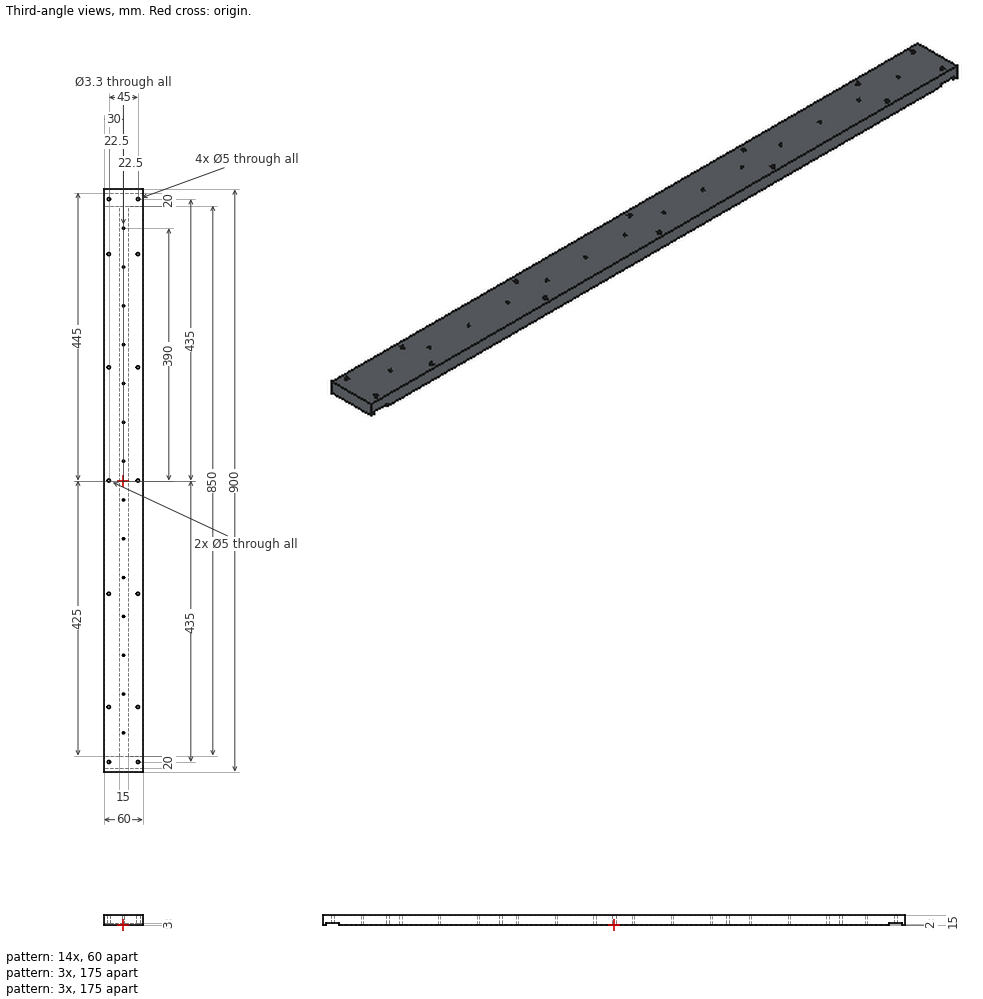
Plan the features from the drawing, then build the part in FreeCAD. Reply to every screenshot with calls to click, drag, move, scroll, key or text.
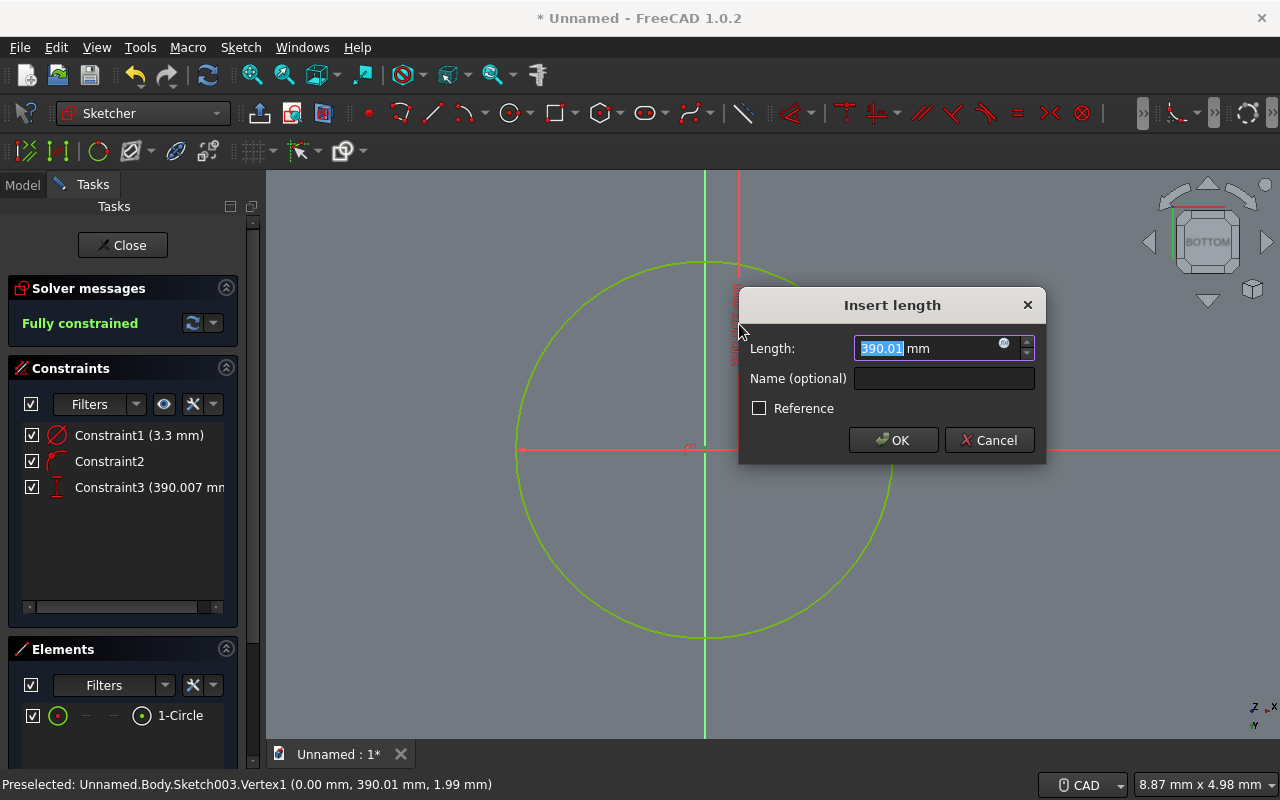
text(390)
key(Return)
key(Escape)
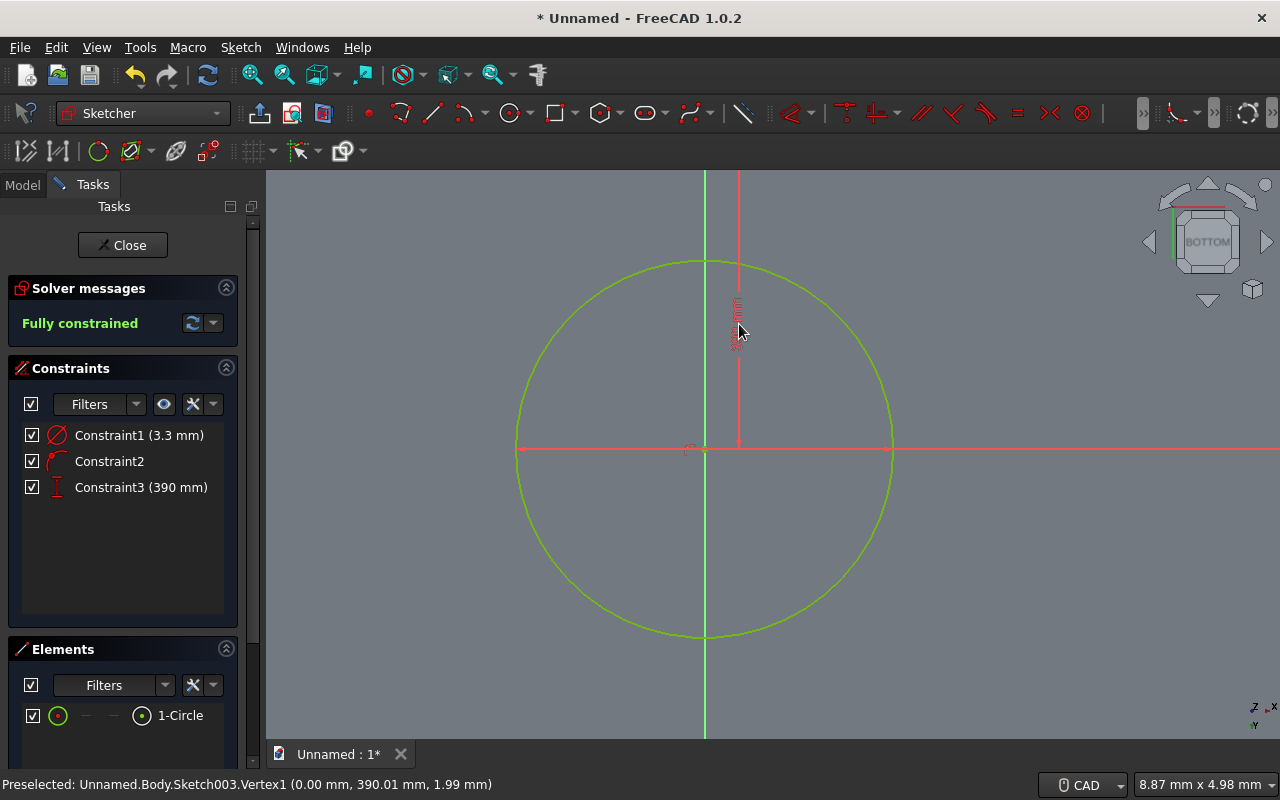
click(123, 245)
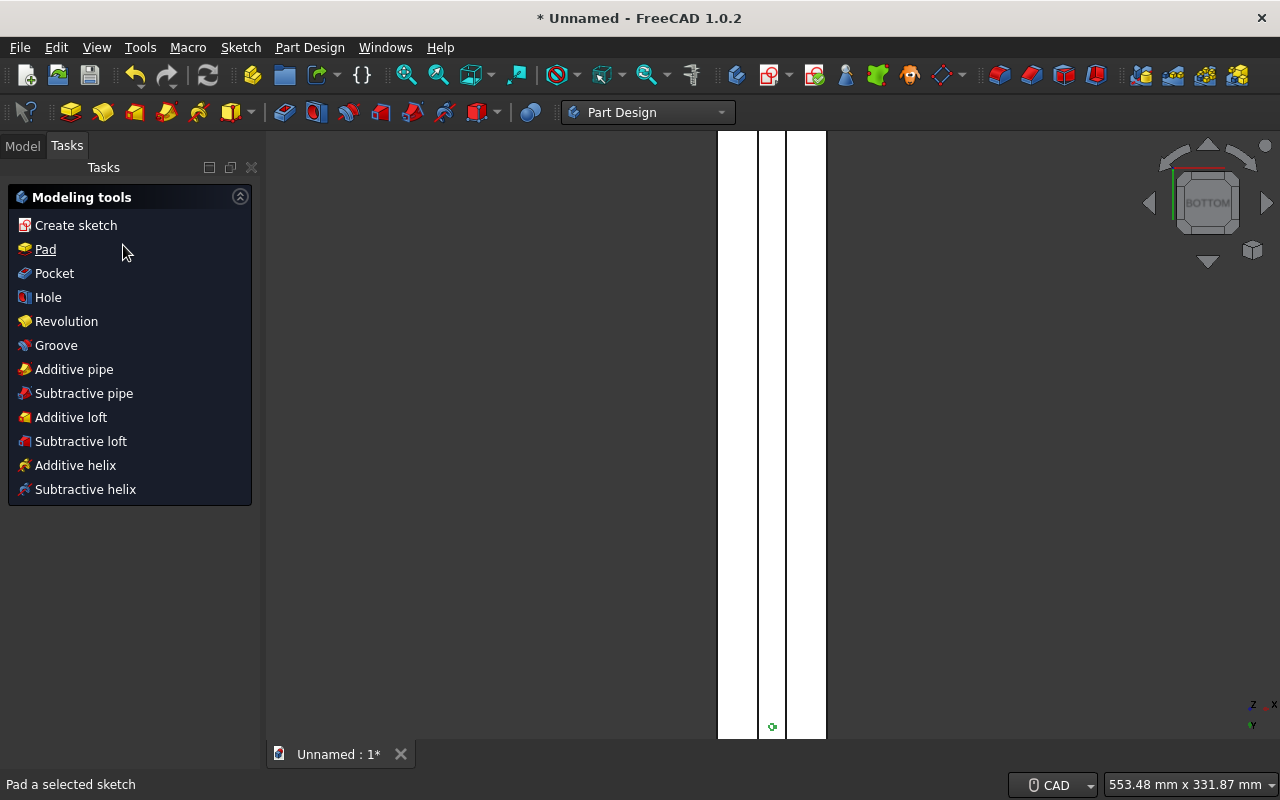
click(318, 112)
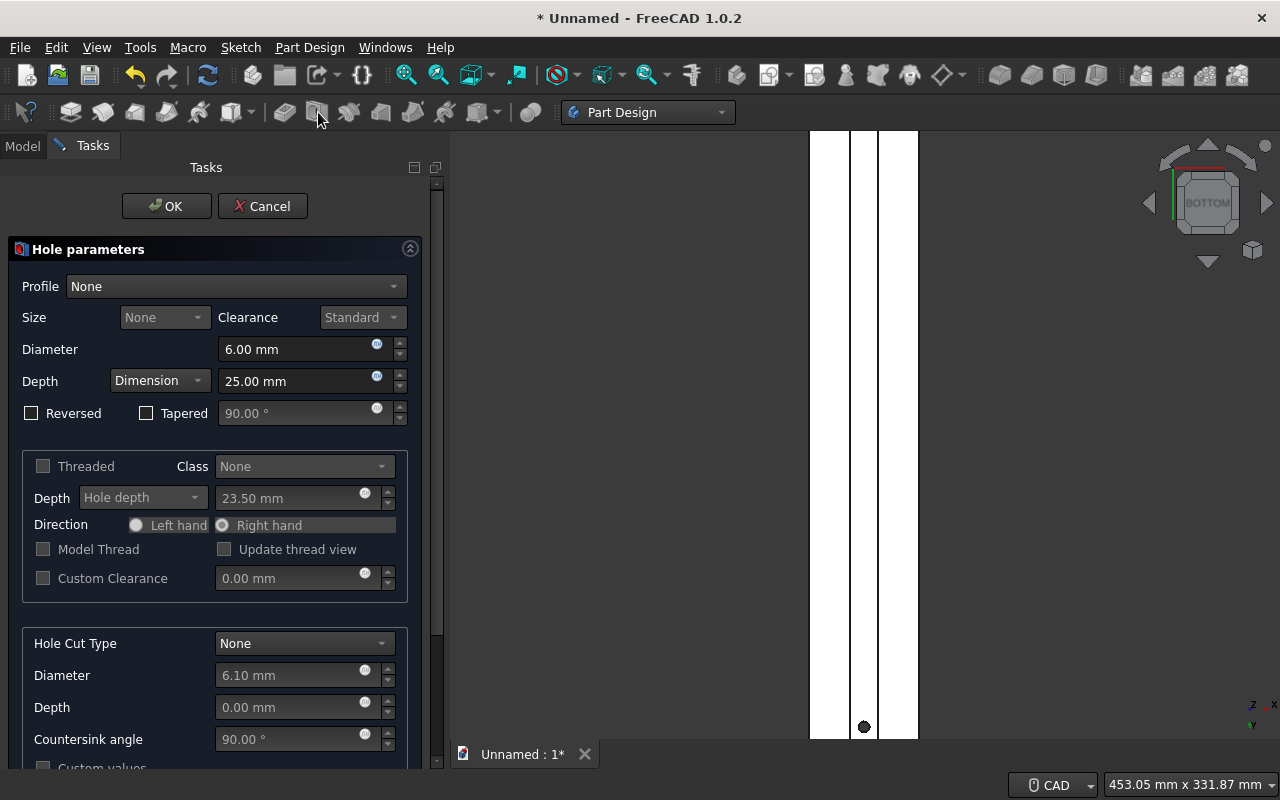
triple_click(305, 349)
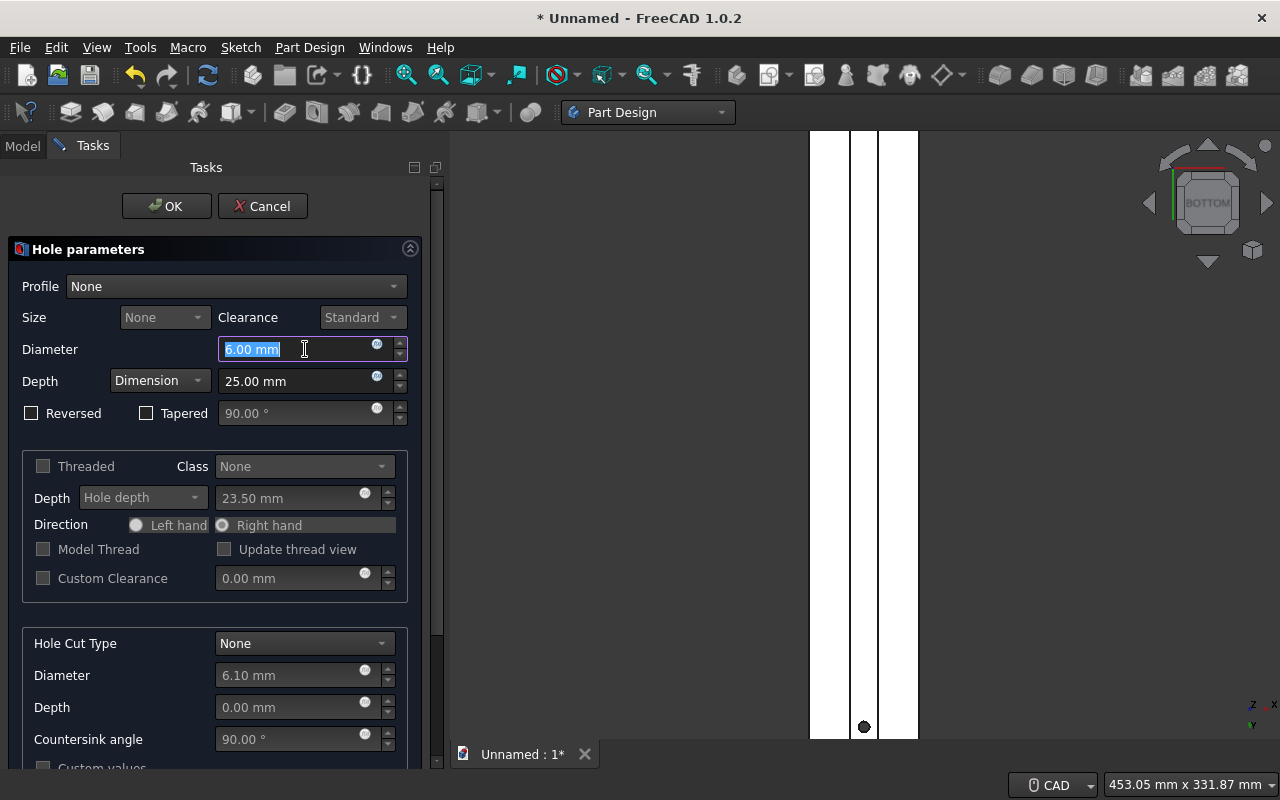
text(3.3)
key(Tab)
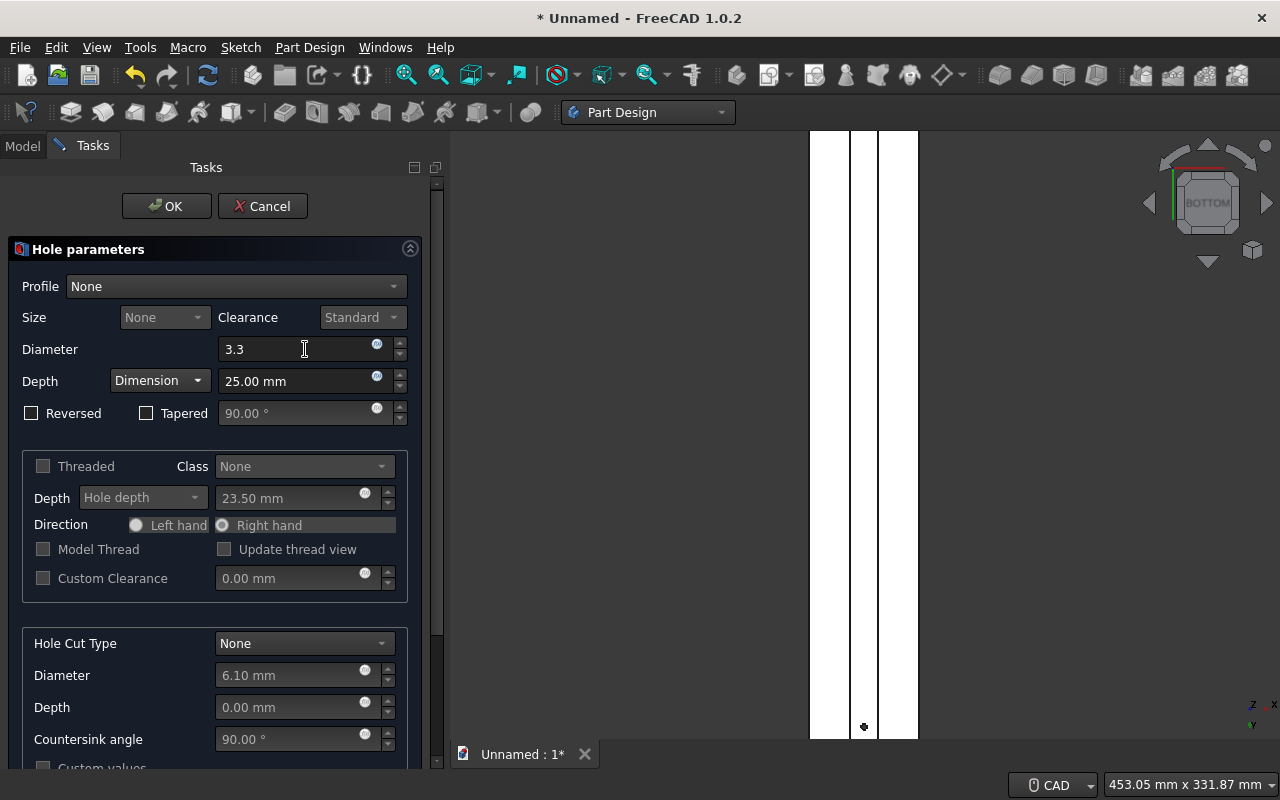
click(161, 380)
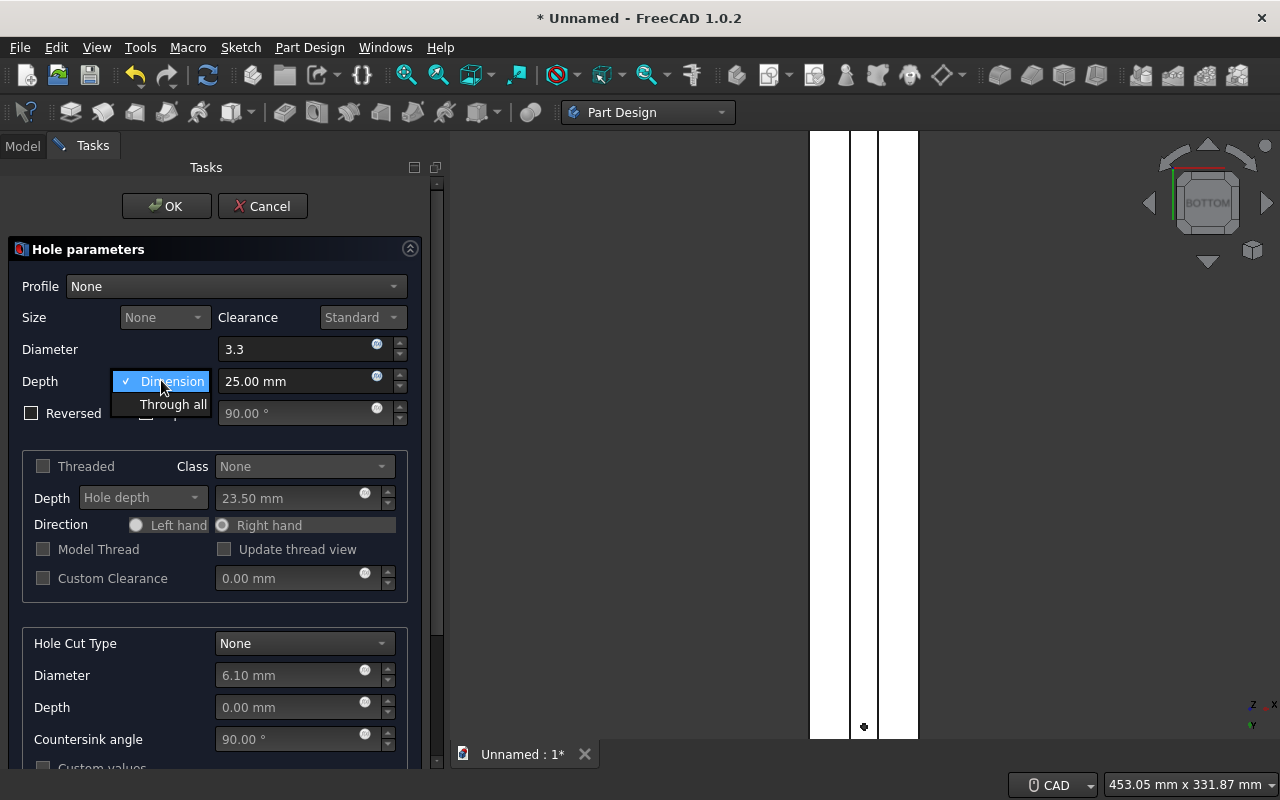
click(160, 404)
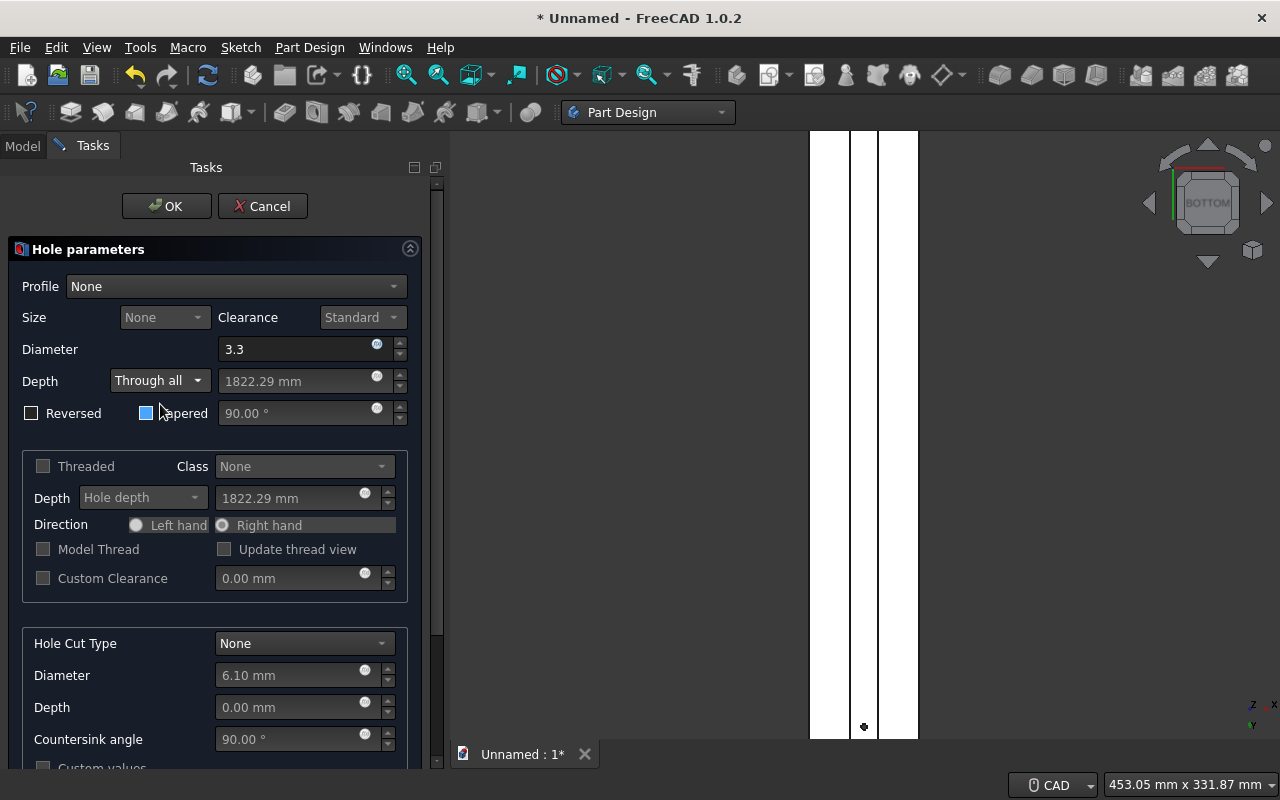
click(167, 206)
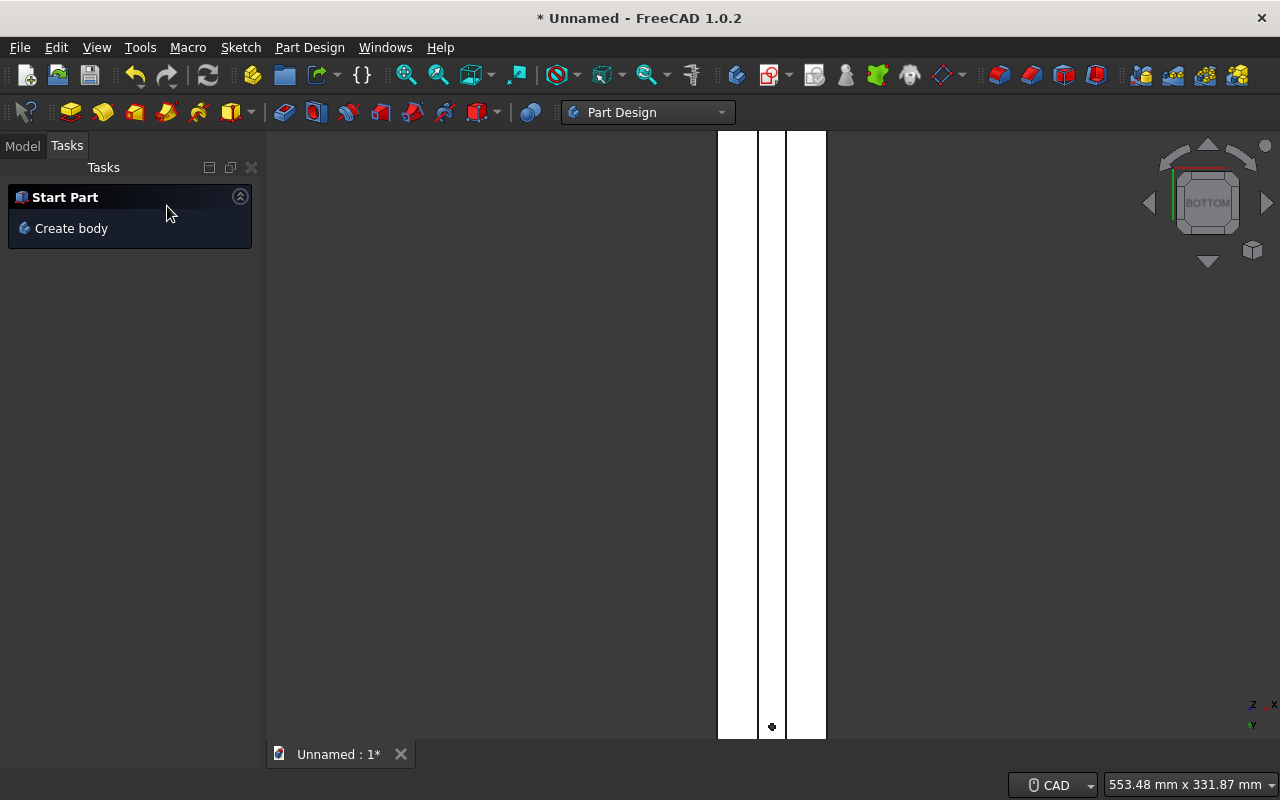
key(v)
key(f)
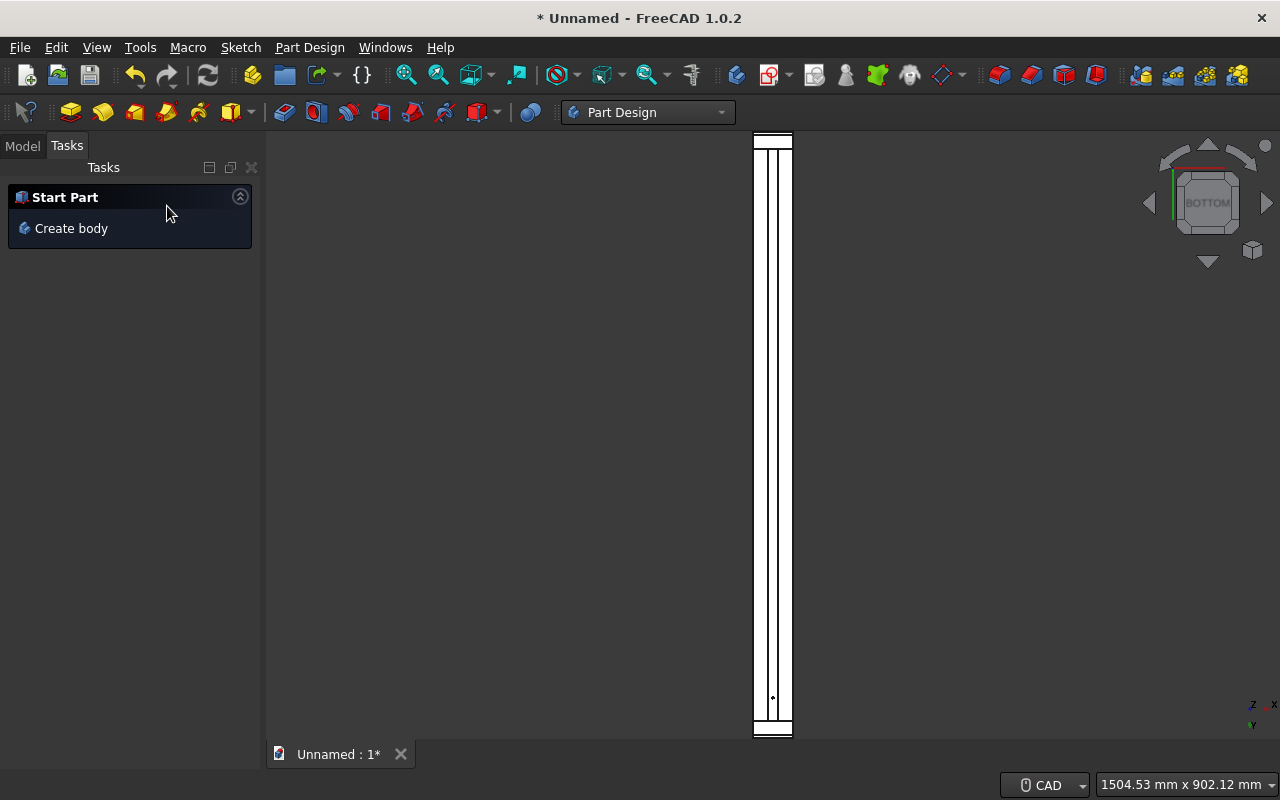
click(23, 145)